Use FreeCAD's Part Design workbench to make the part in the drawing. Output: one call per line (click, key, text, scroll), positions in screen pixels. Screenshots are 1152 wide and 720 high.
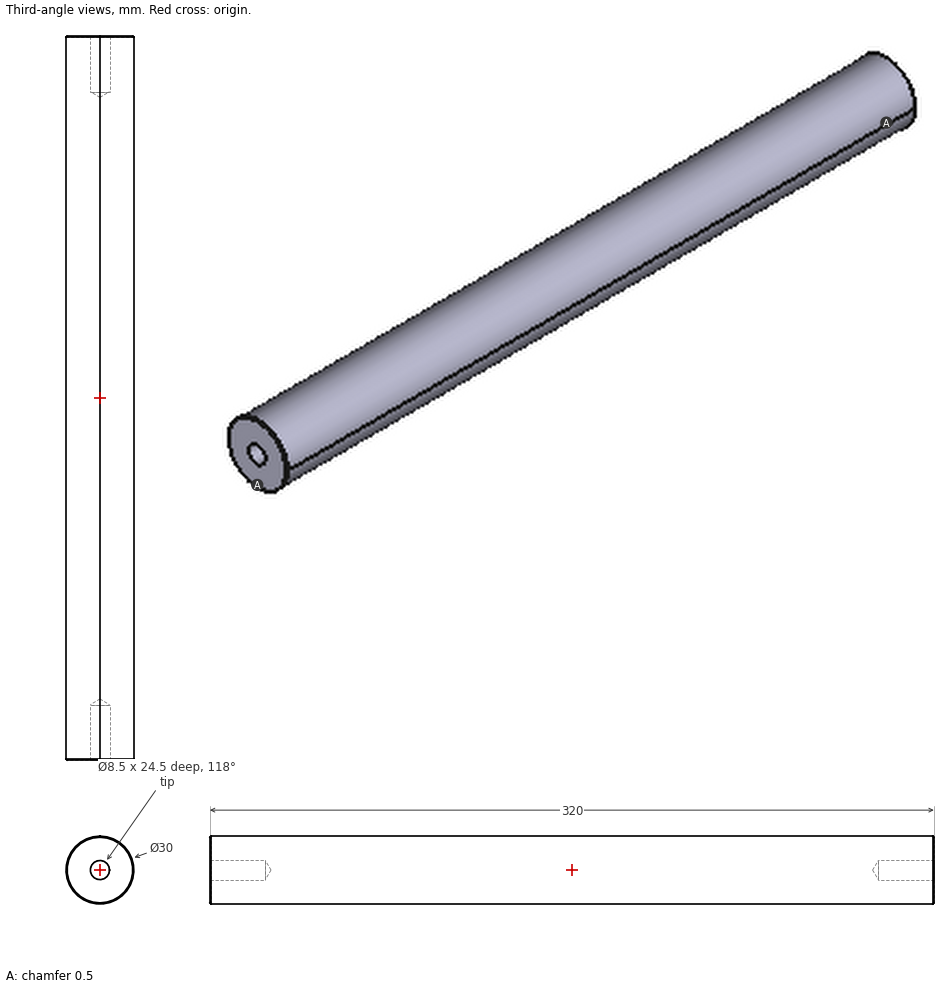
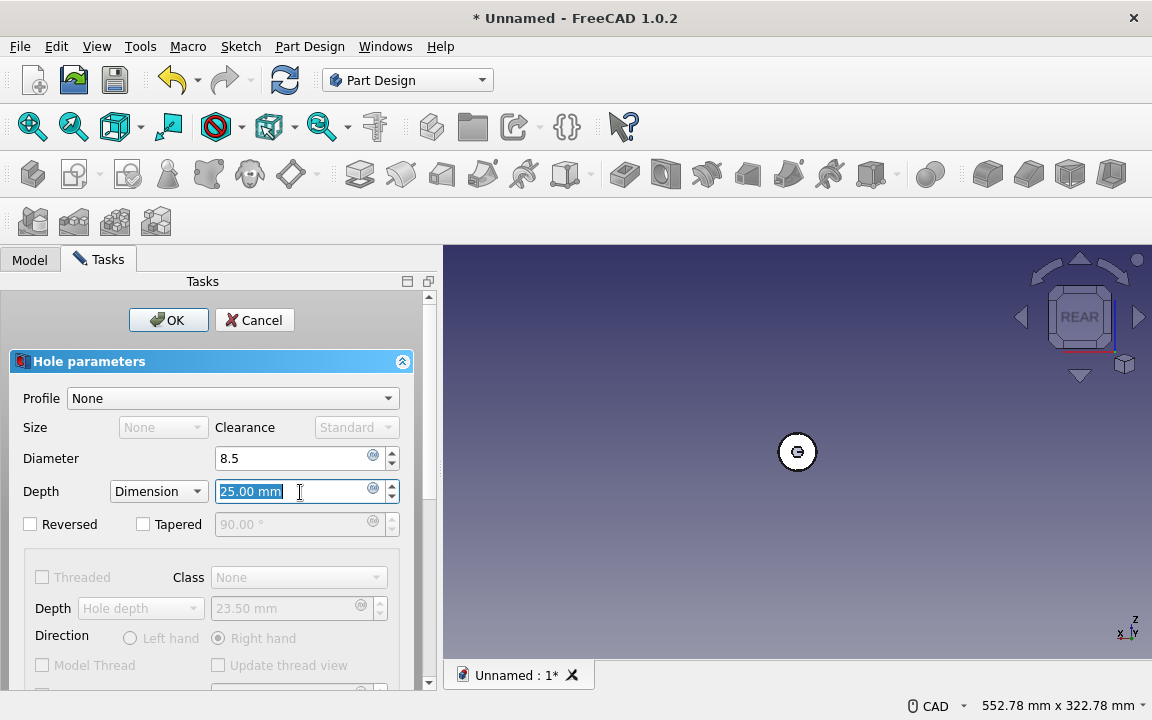
text(24.5)
key(Tab)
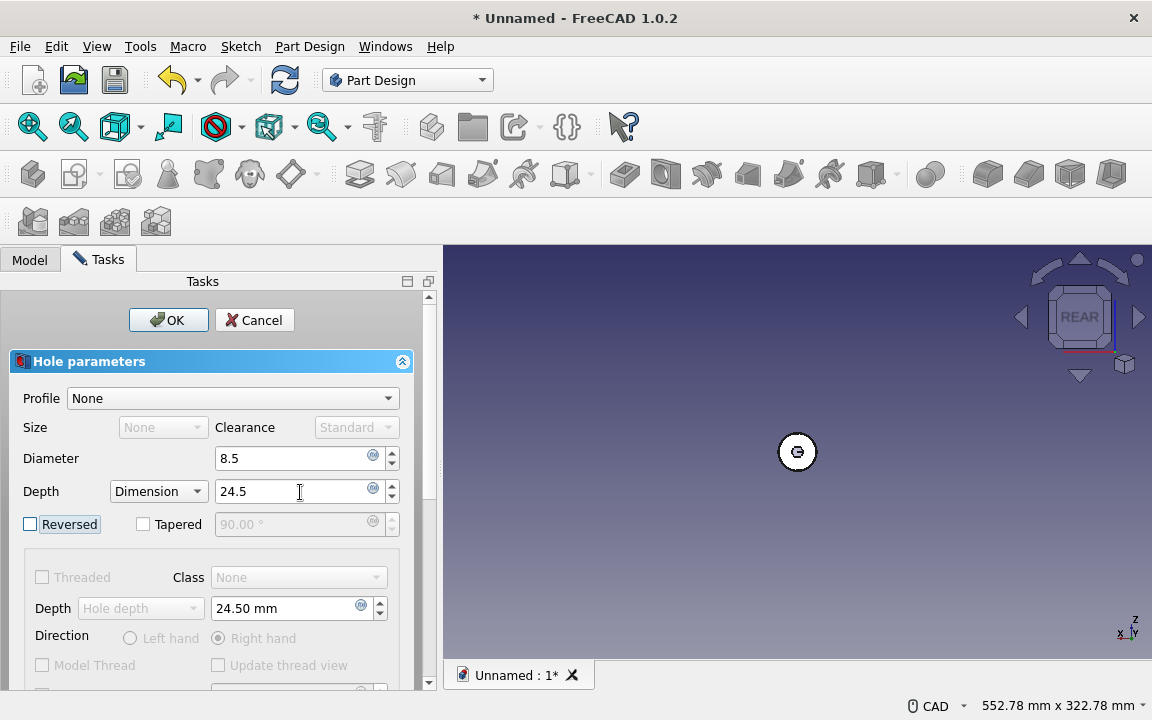
click(169, 320)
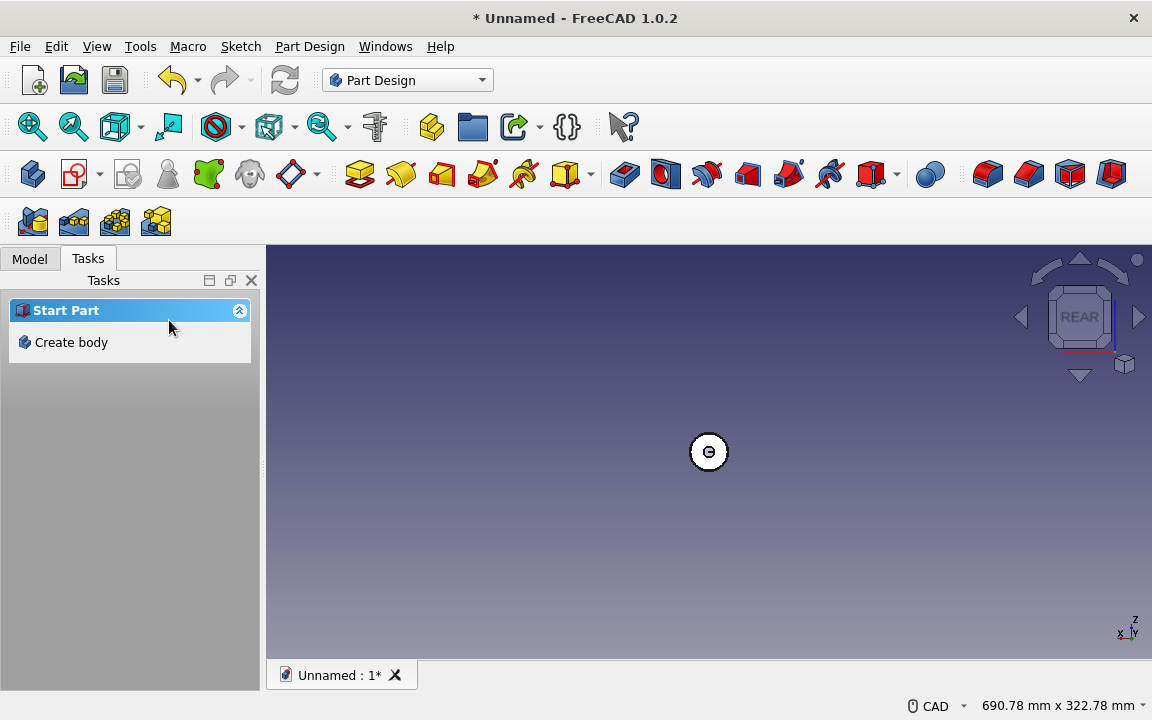
key(v)
key(f)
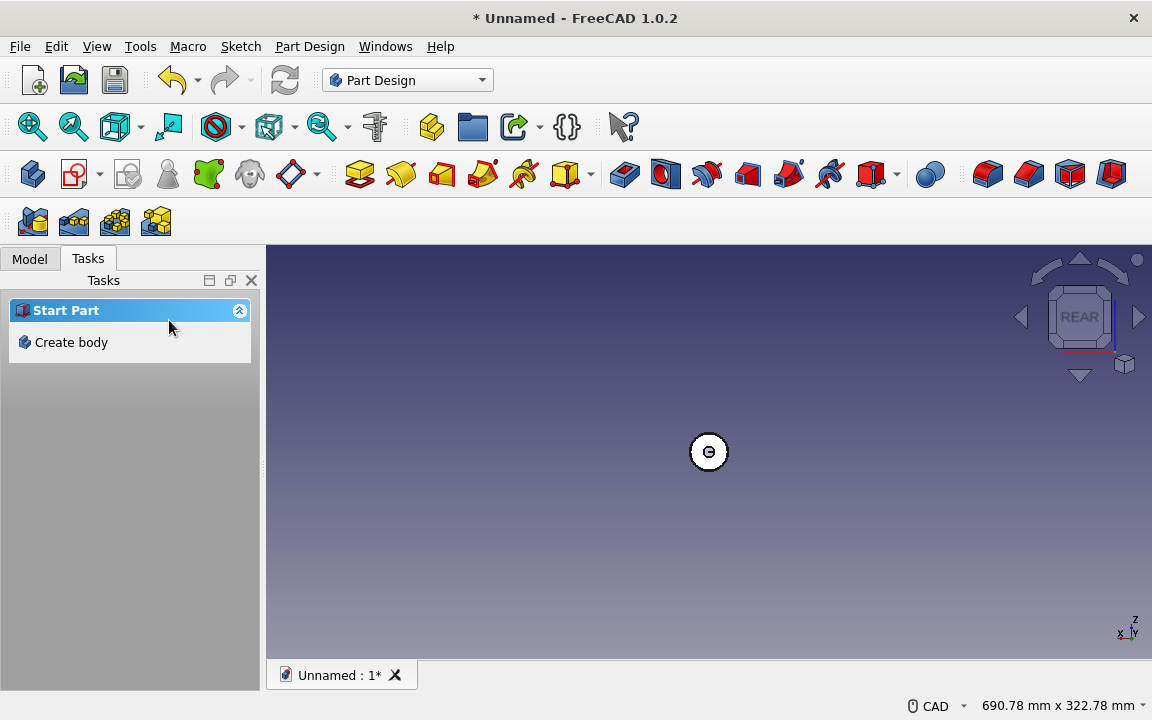
key(0)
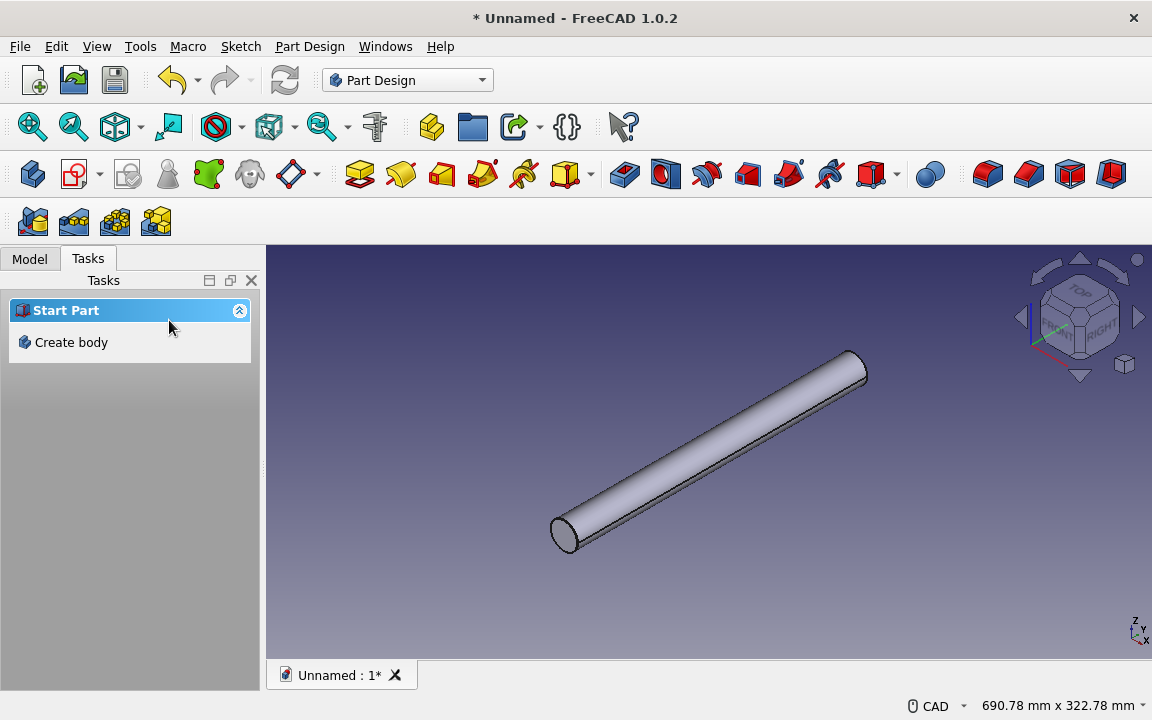
click(564, 535)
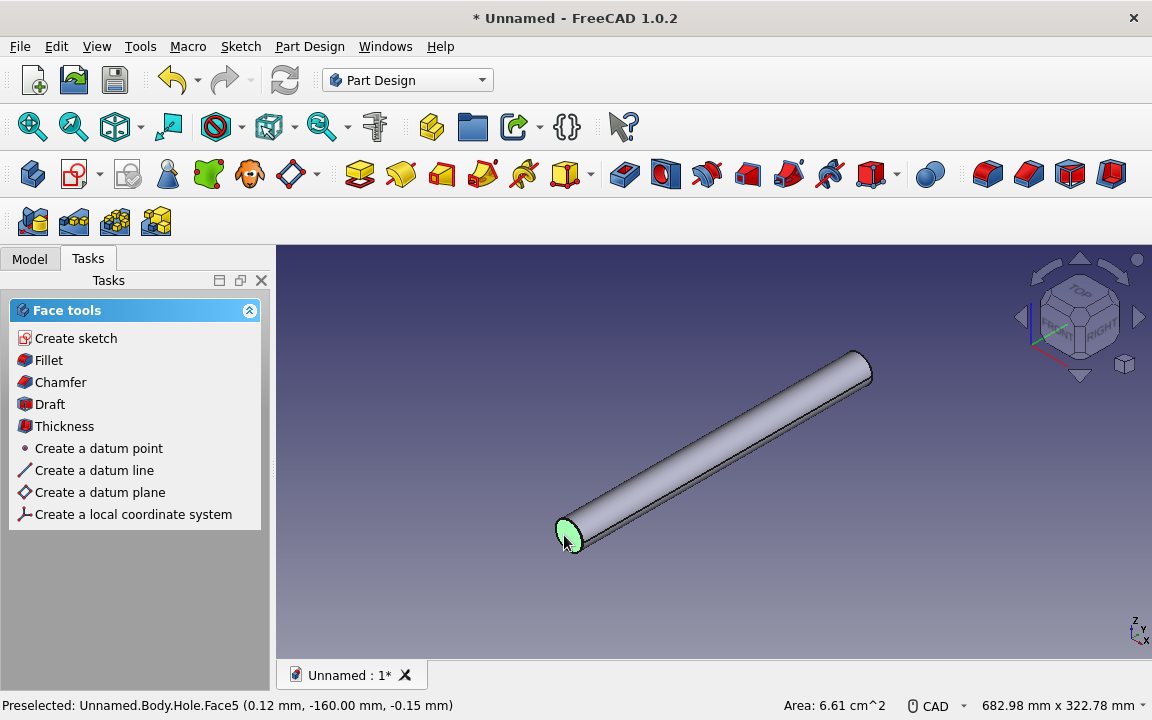
click(74, 174)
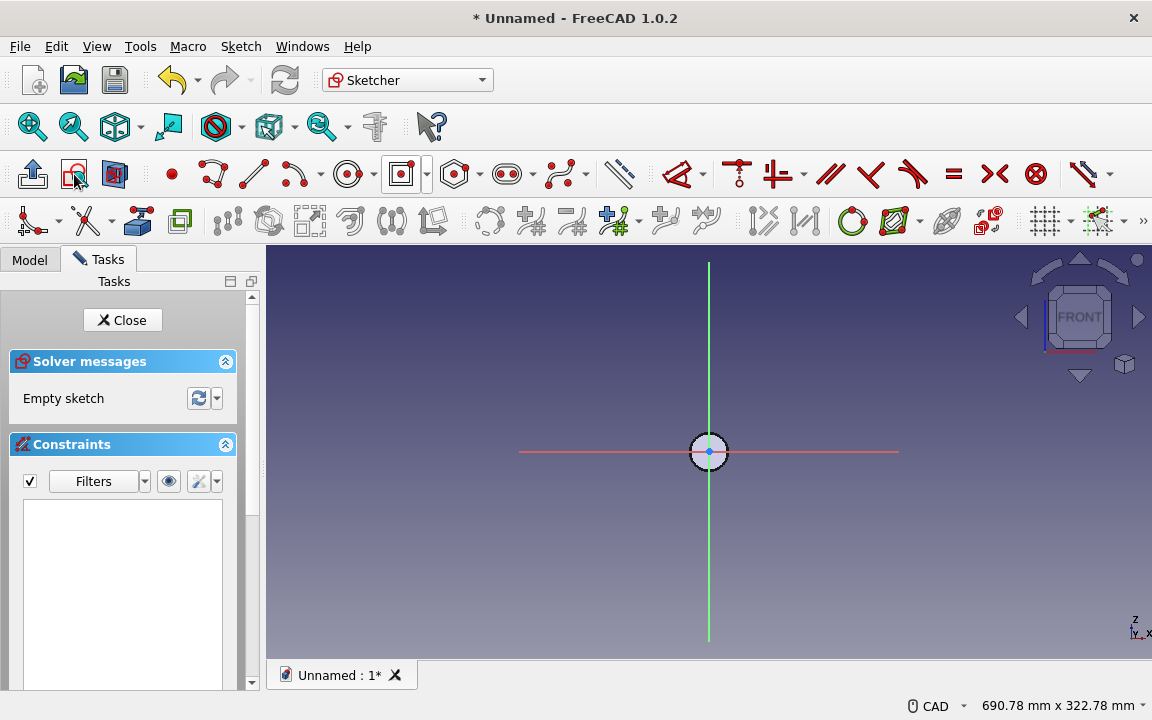
scroll(713, 452, up, 15)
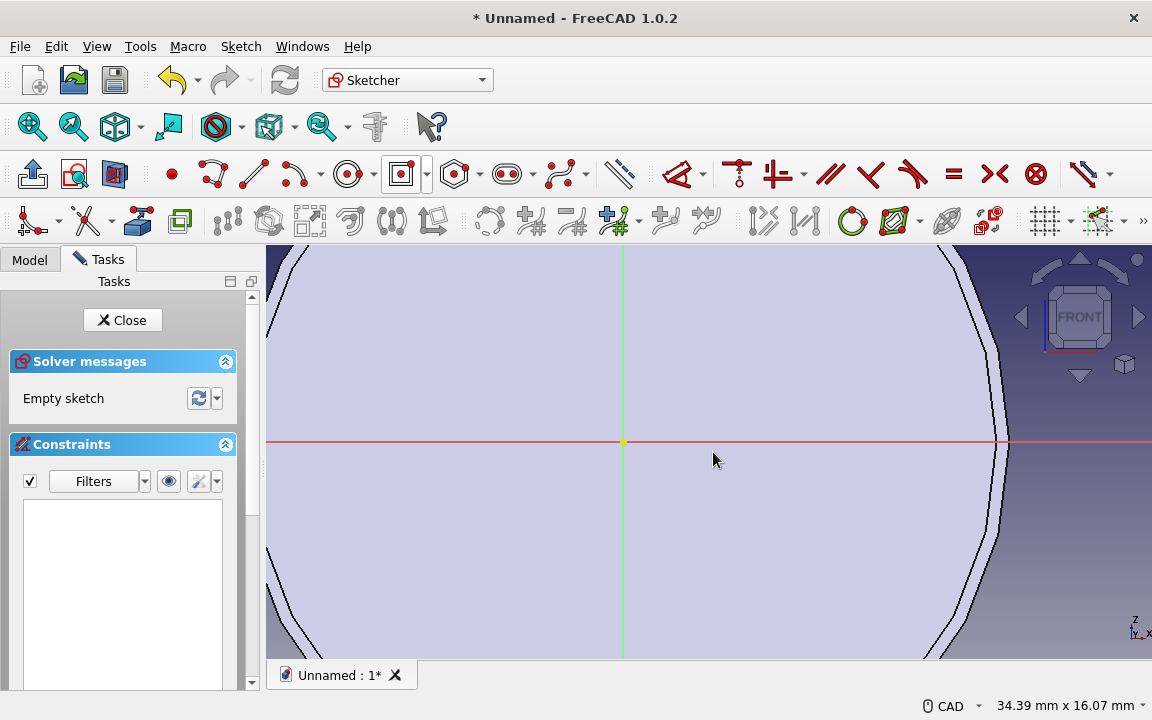
click(348, 174)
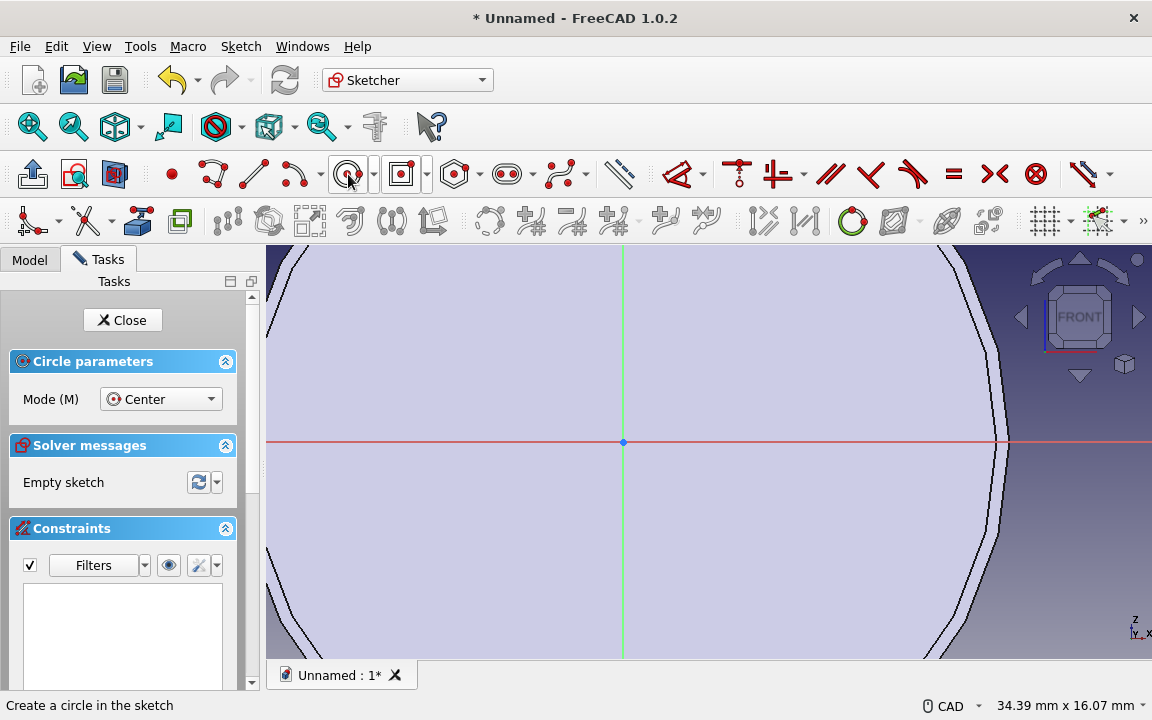
click(623, 442)
click(700, 365)
key(Escape)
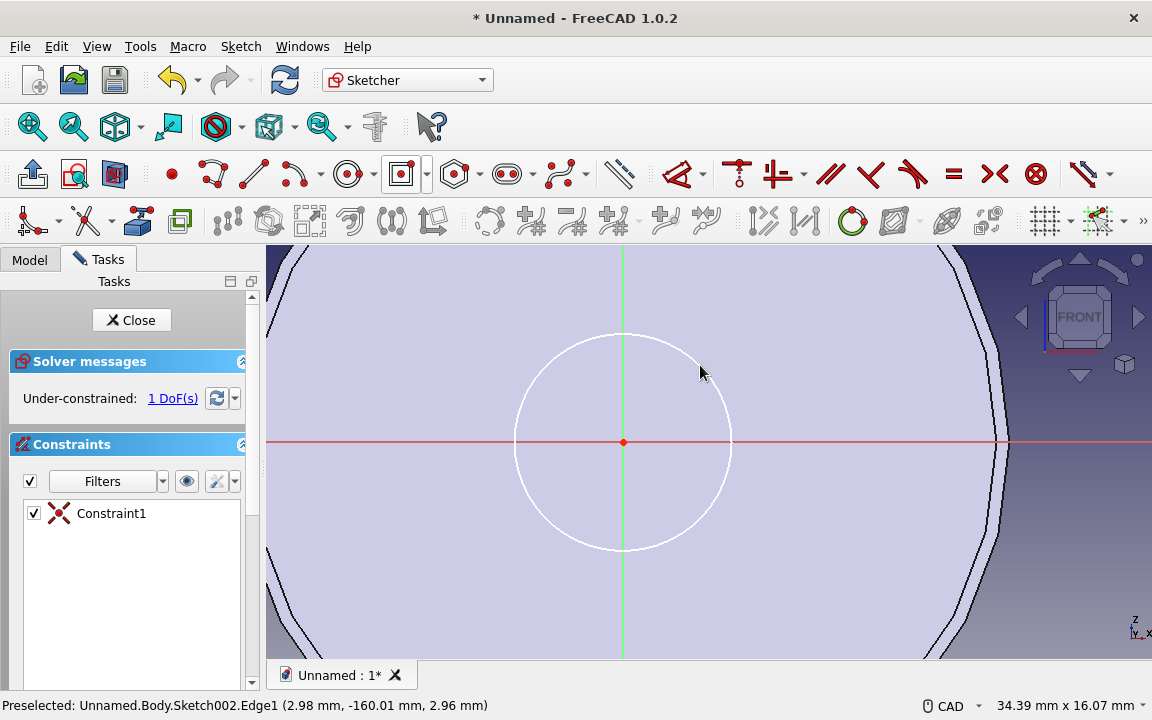
click(699, 365)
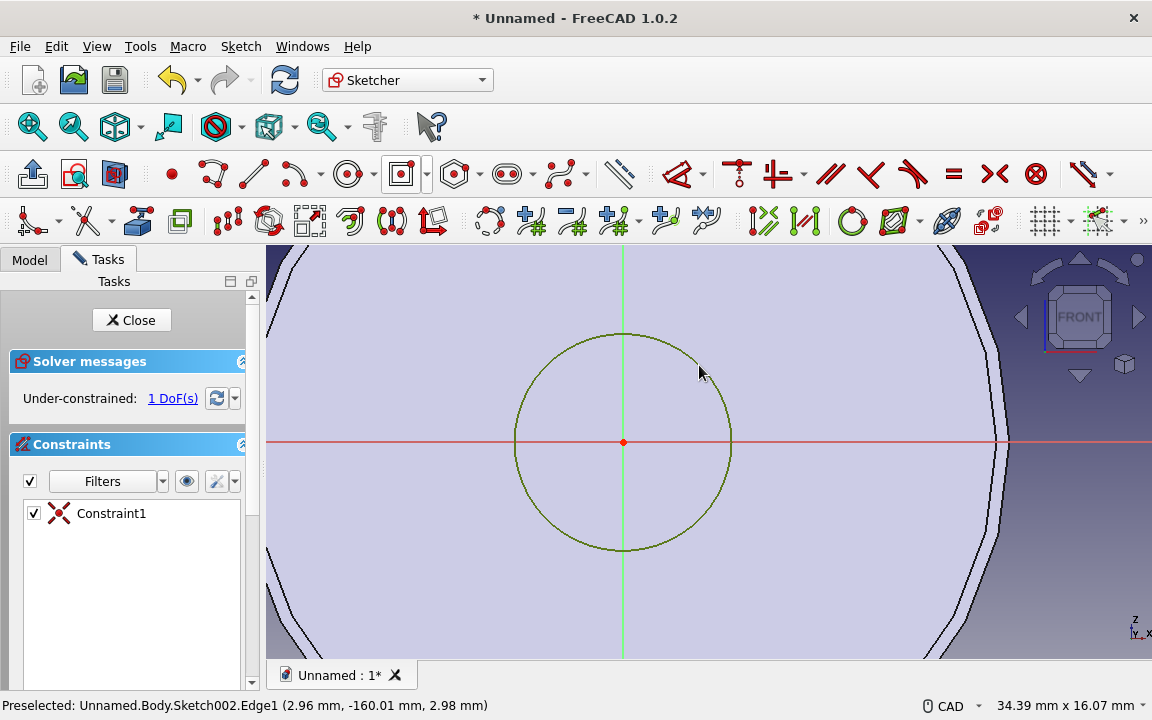
key(k)
key(o)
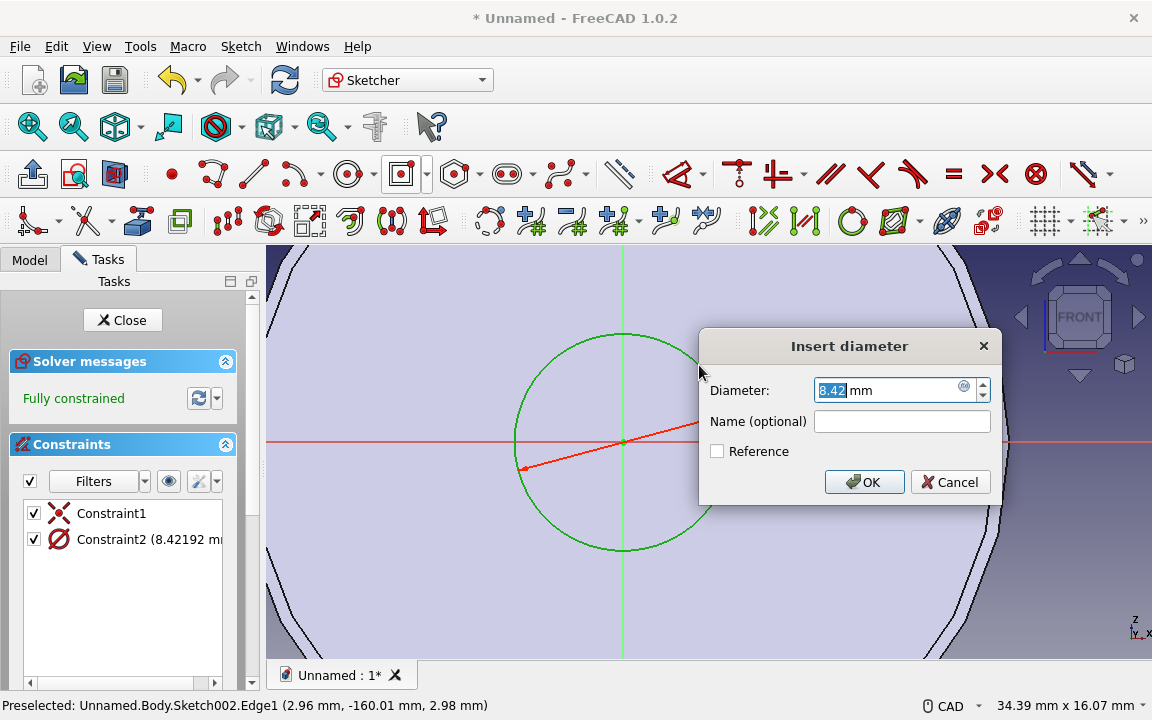
text(8.5)
key(Return)